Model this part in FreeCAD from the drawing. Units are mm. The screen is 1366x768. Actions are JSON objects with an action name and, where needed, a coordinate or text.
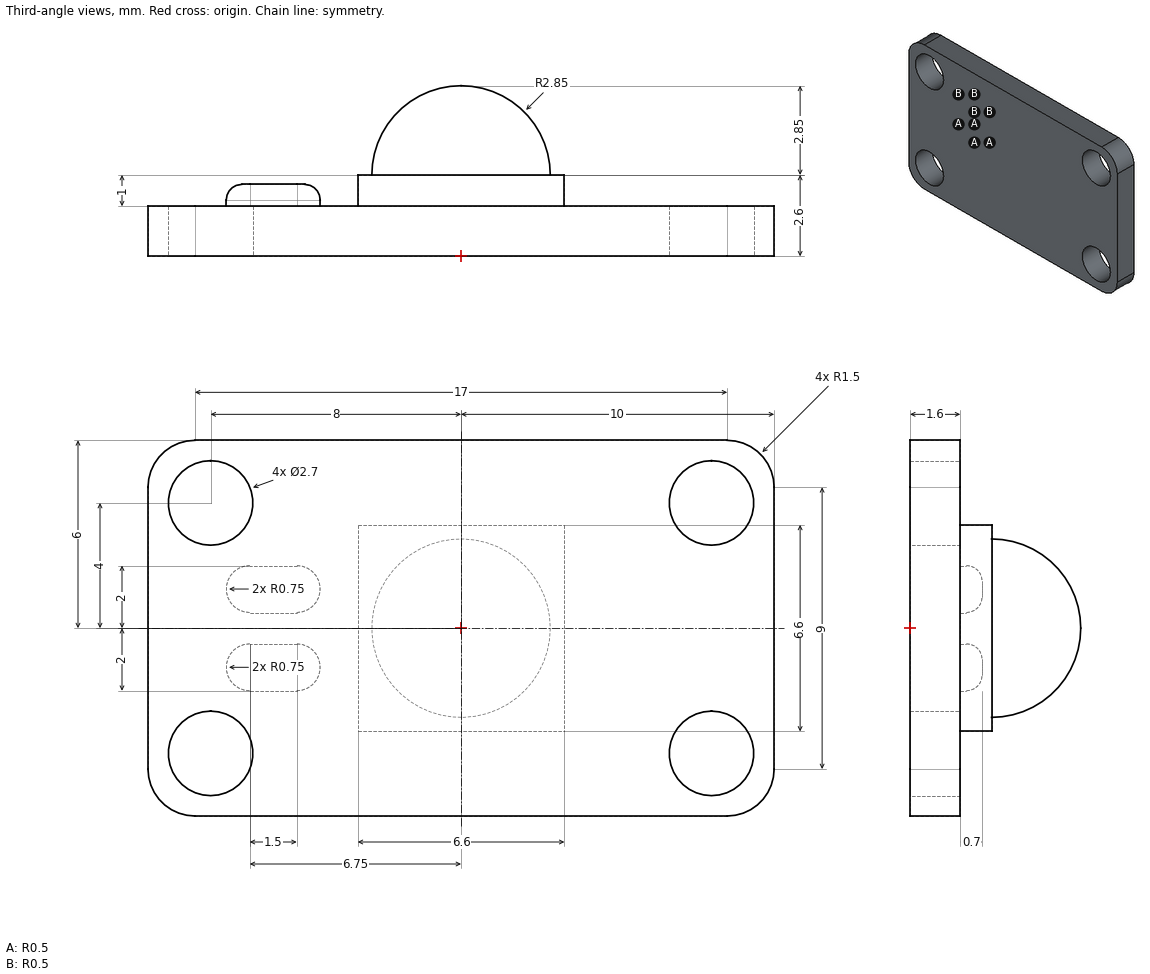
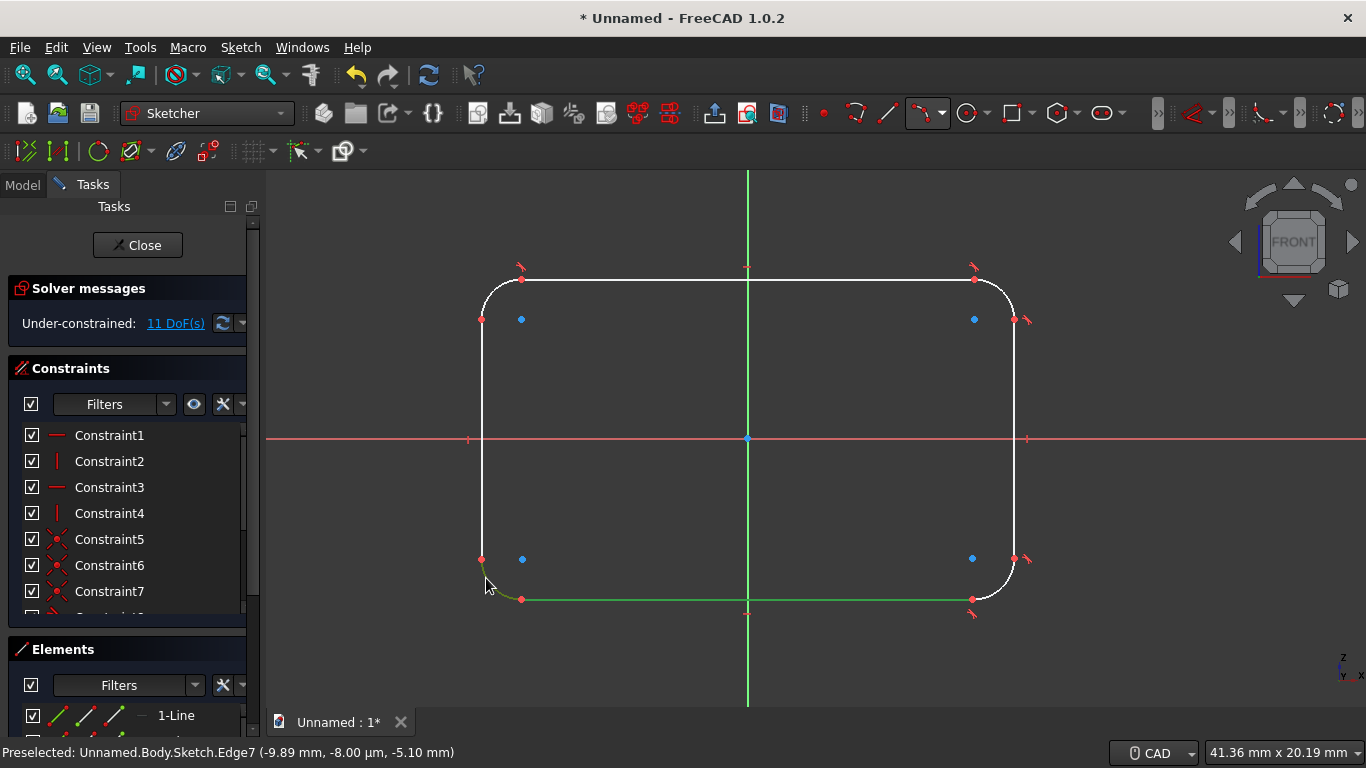
{"action": "key", "text": "t"}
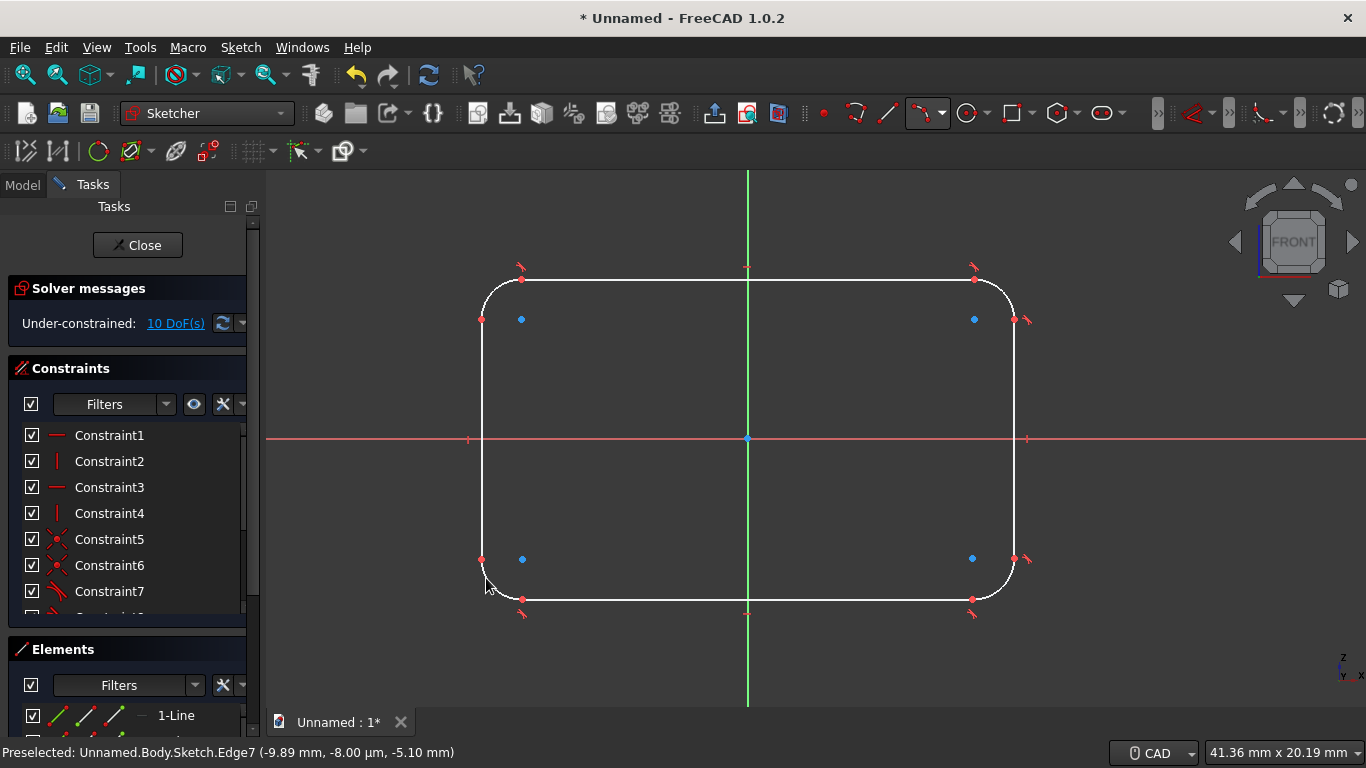
{"action": "left_click", "coordinate": [482, 487]}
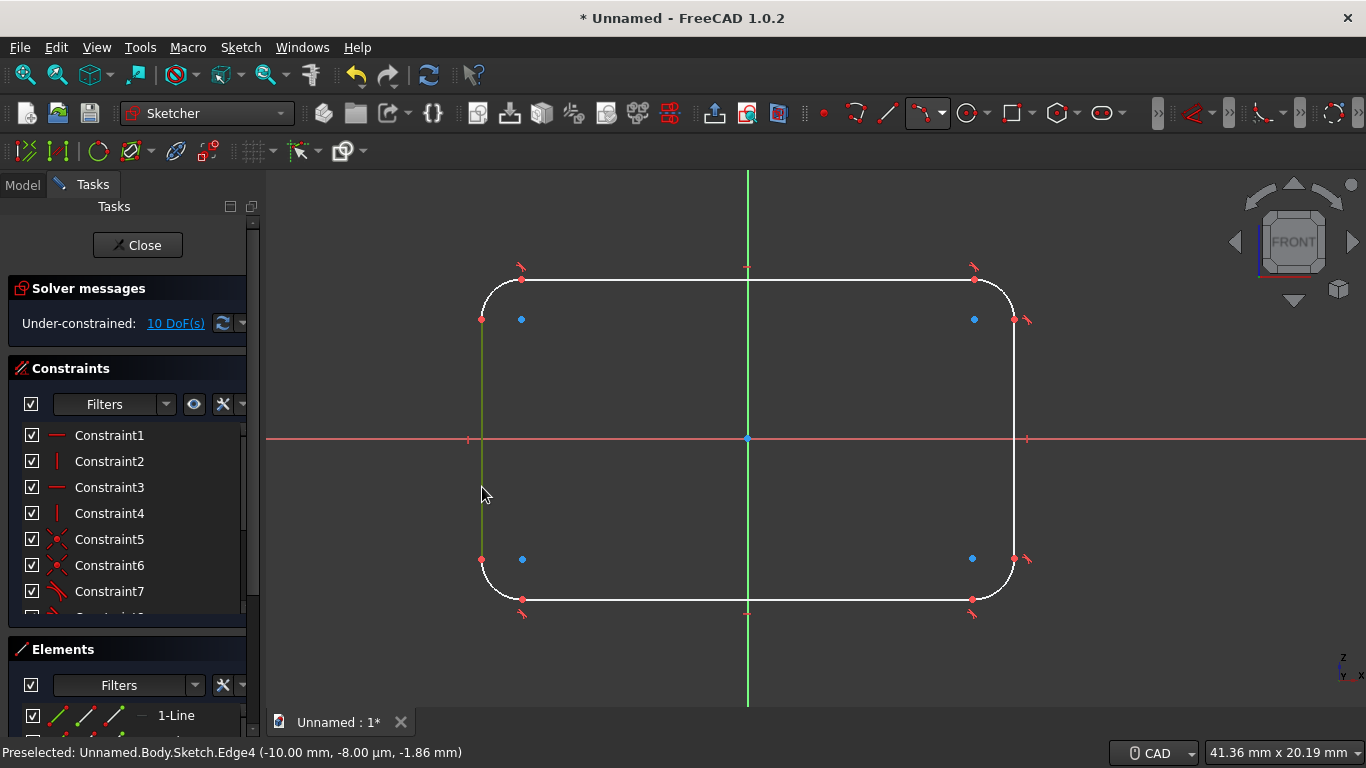
{"action": "left_click", "coordinate": [486, 578]}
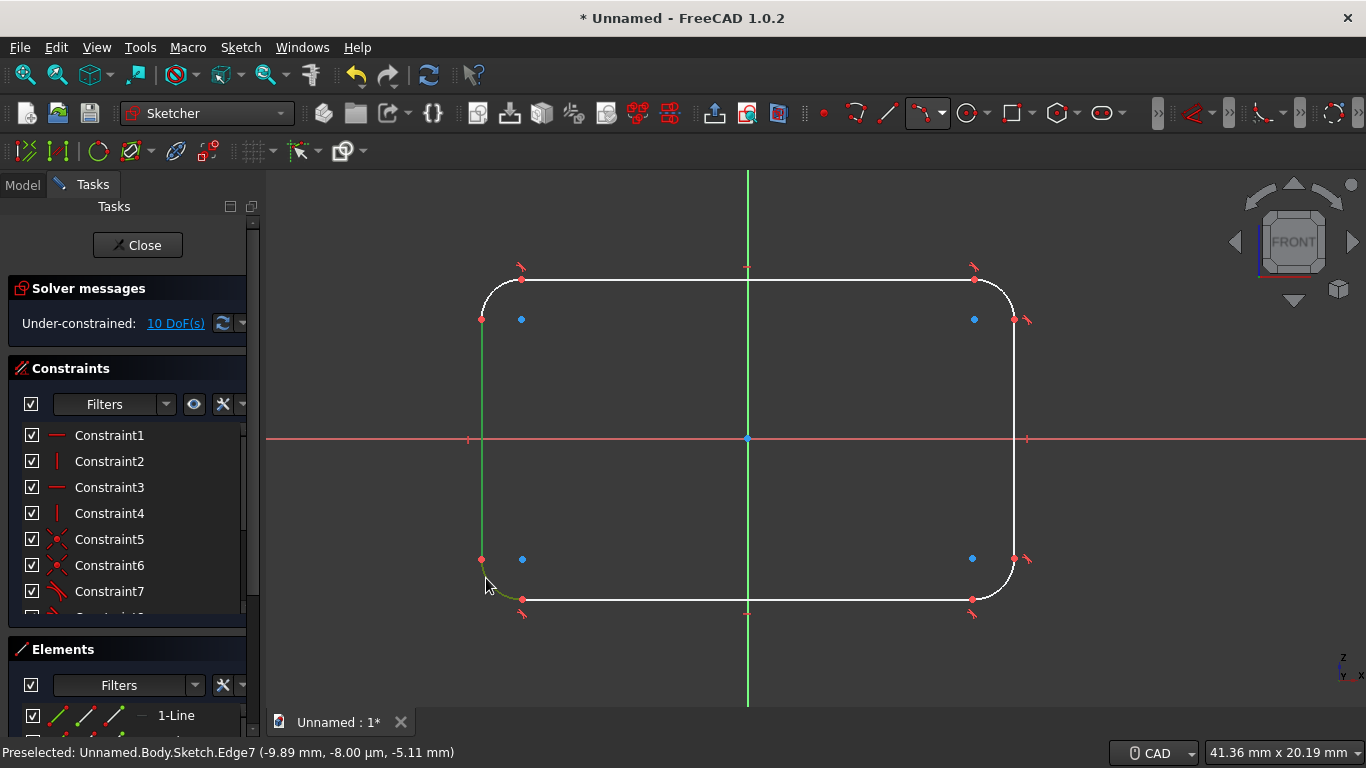
{"action": "key", "text": "t"}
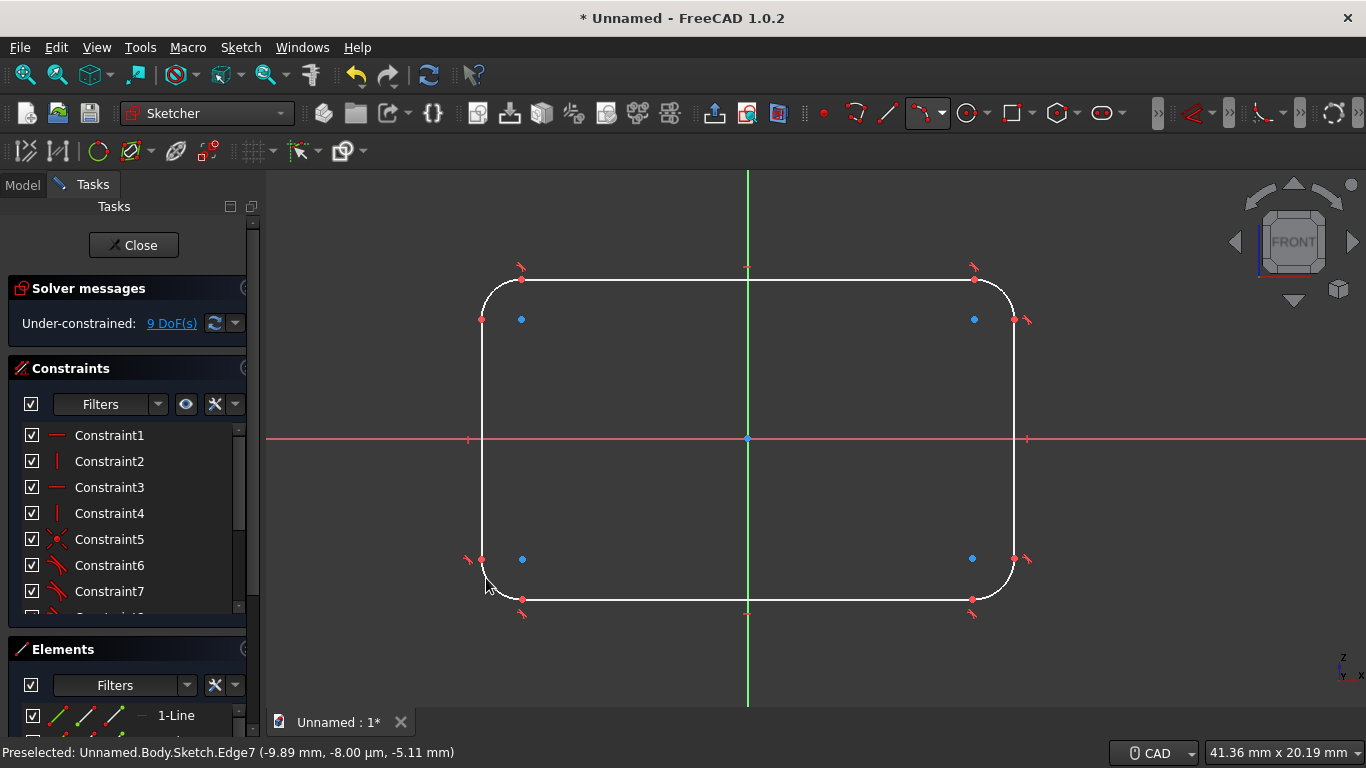
{"action": "left_click", "coordinate": [482, 487]}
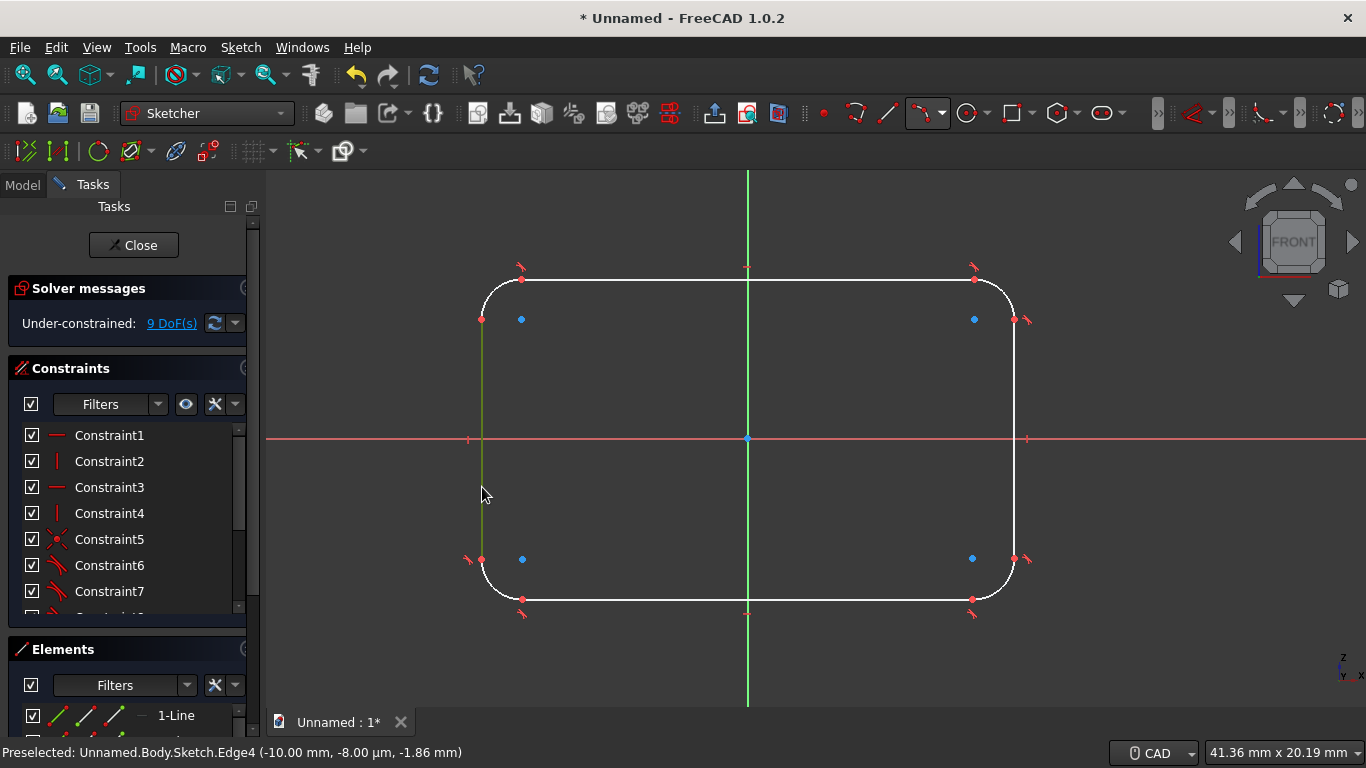
{"action": "left_click", "coordinate": [504, 284]}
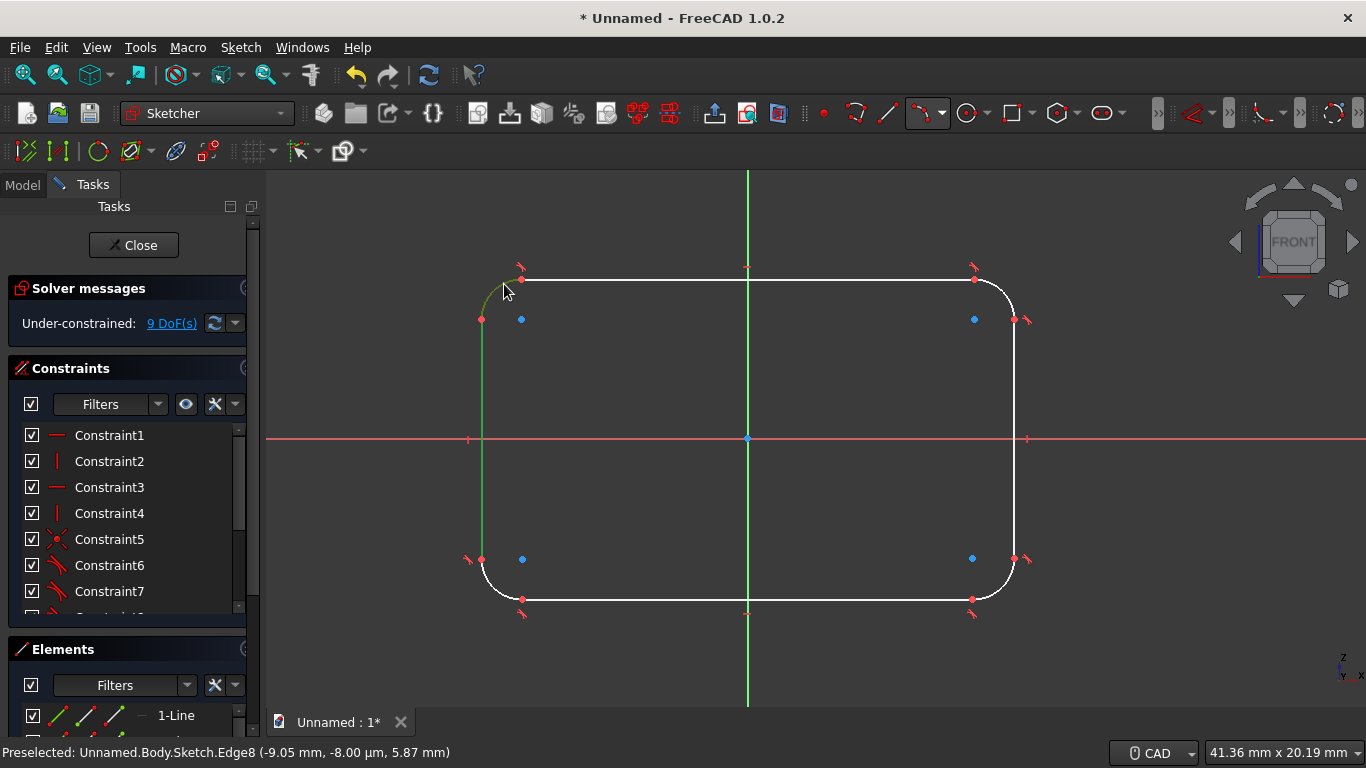
{"action": "key", "text": "t"}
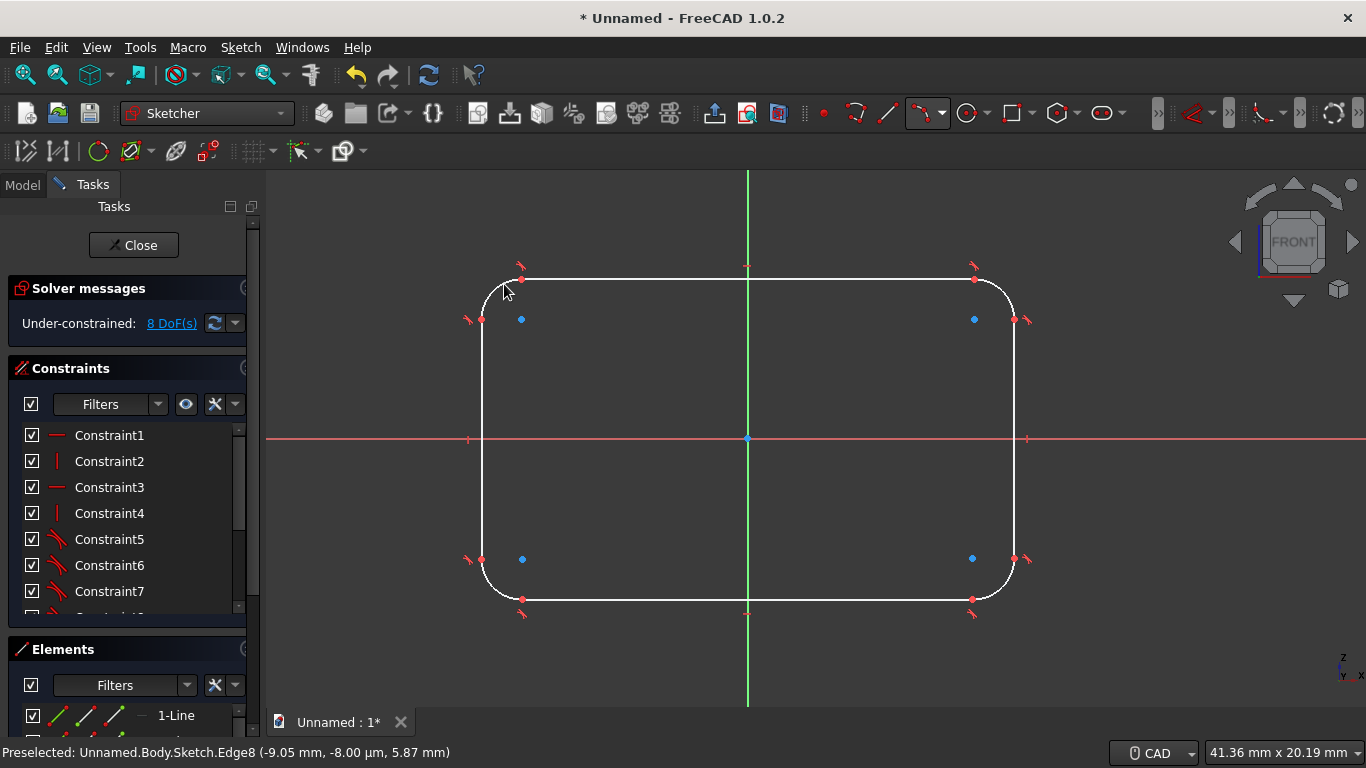
{"action": "left_click", "coordinate": [1010, 301]}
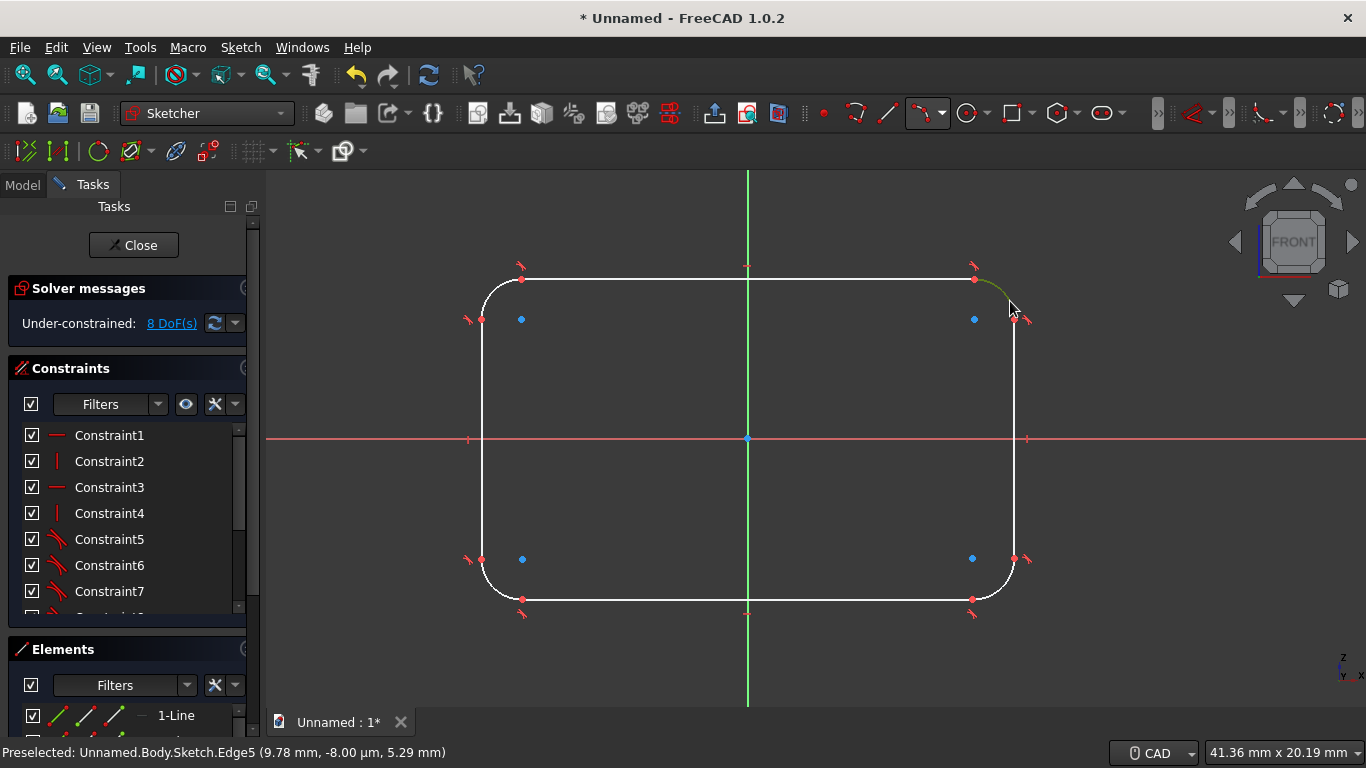
{"action": "left_click", "coordinate": [991, 595]}